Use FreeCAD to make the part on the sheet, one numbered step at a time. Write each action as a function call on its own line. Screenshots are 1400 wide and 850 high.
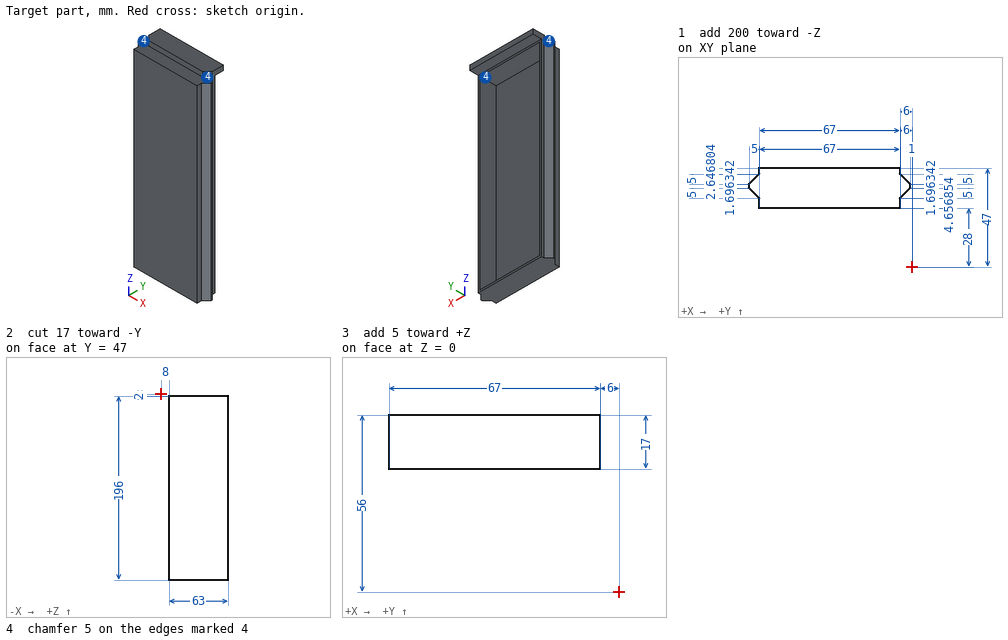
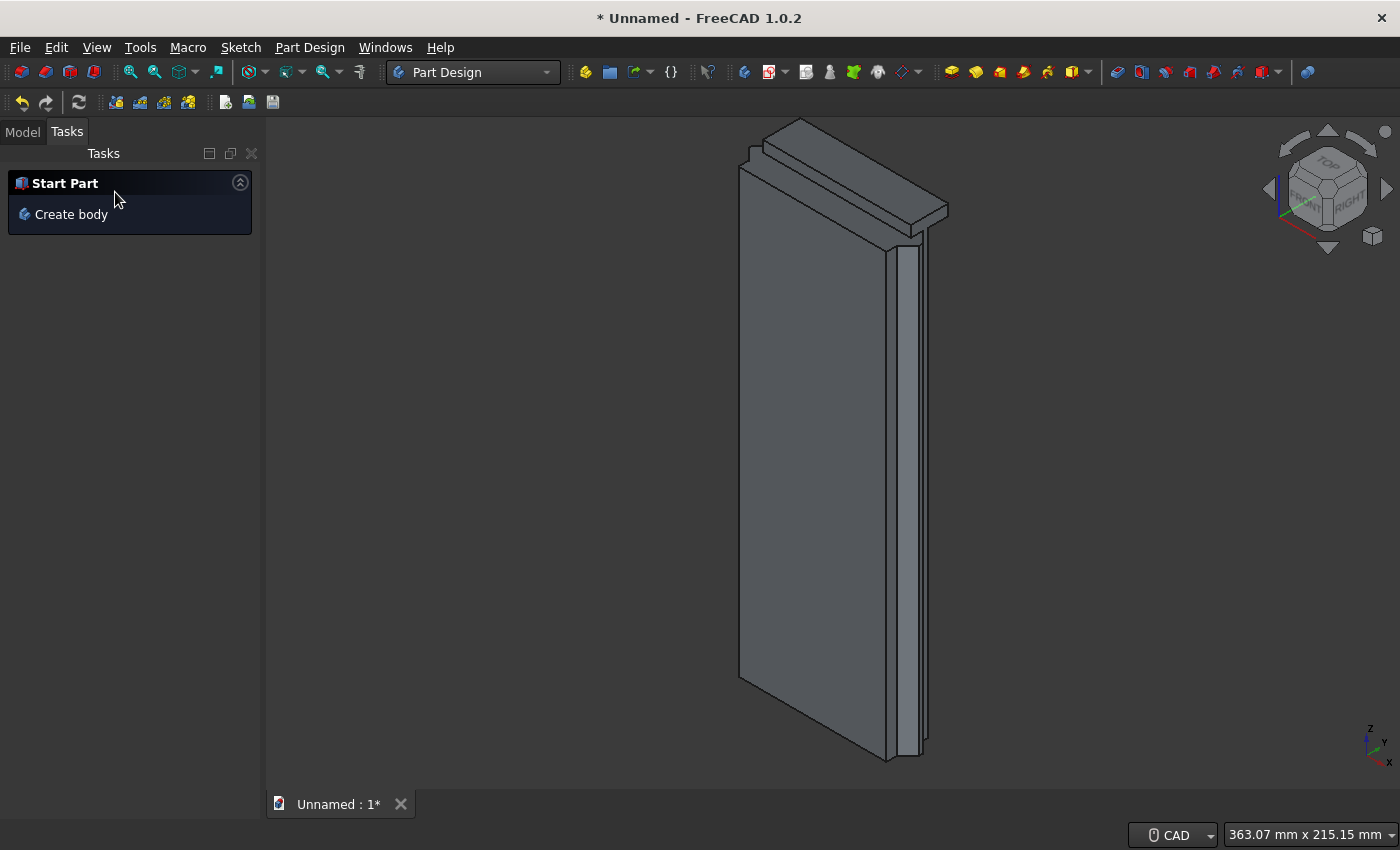
key(v)
key(f)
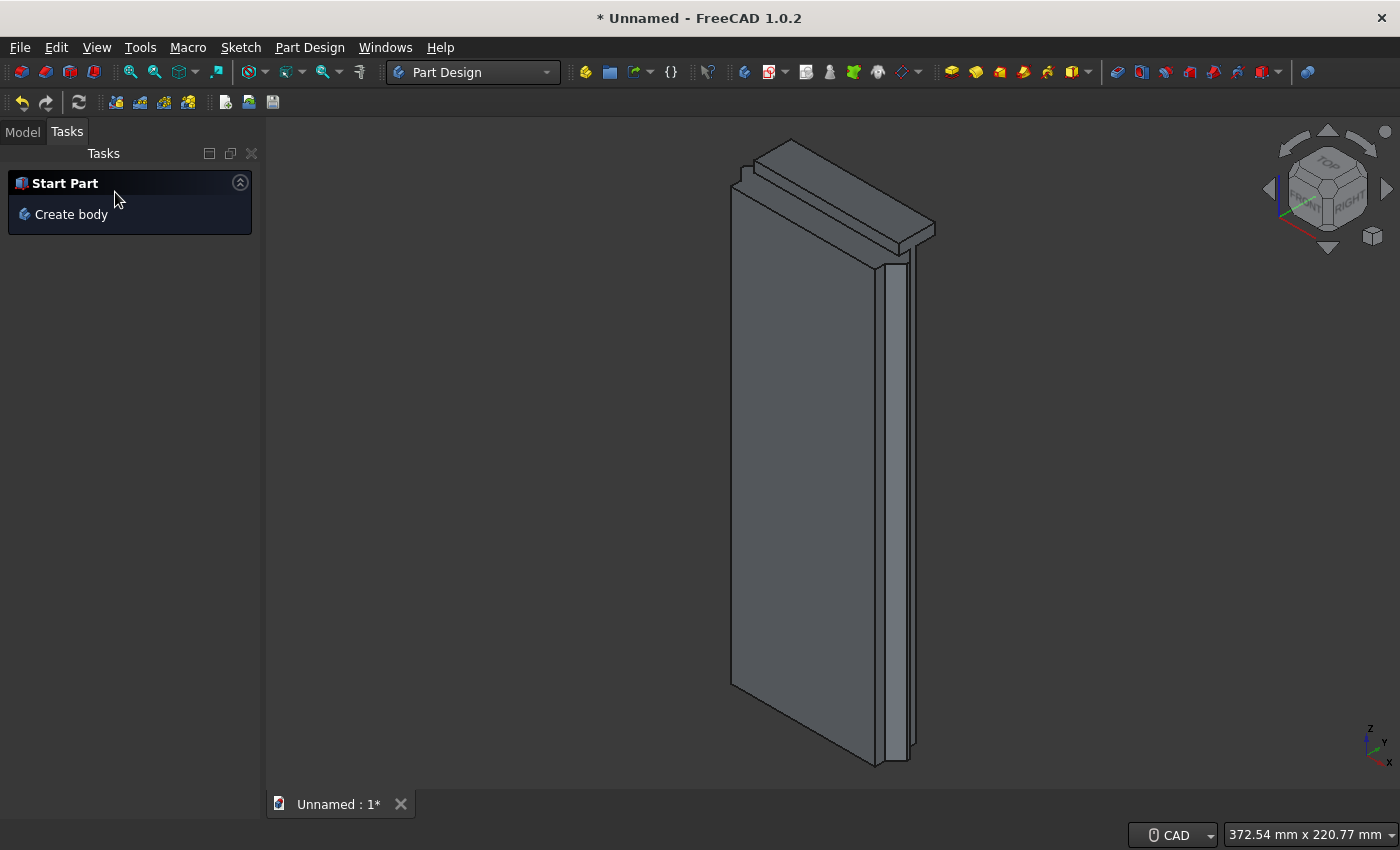
click(899, 249)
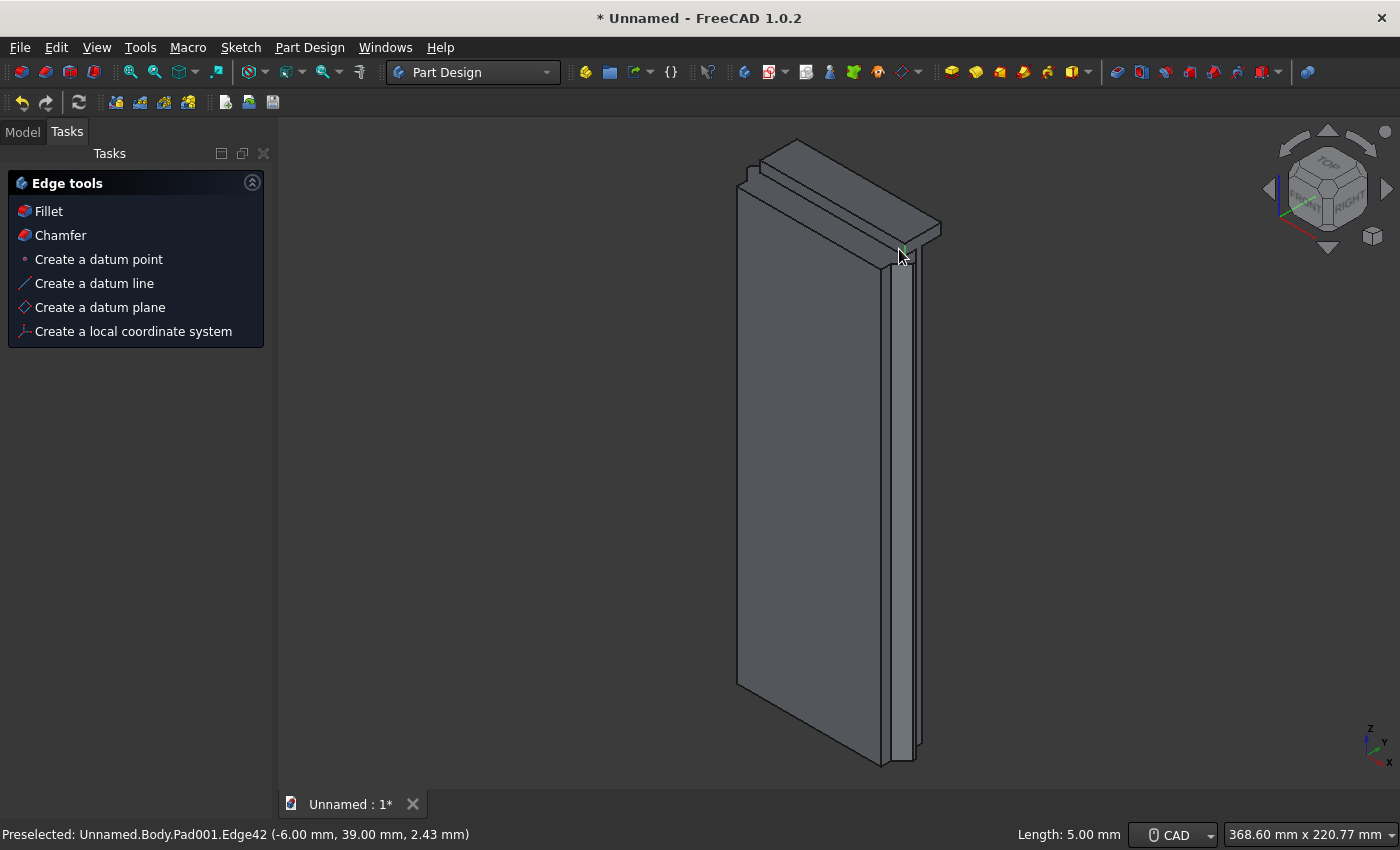
scroll(760, 166, up, 5)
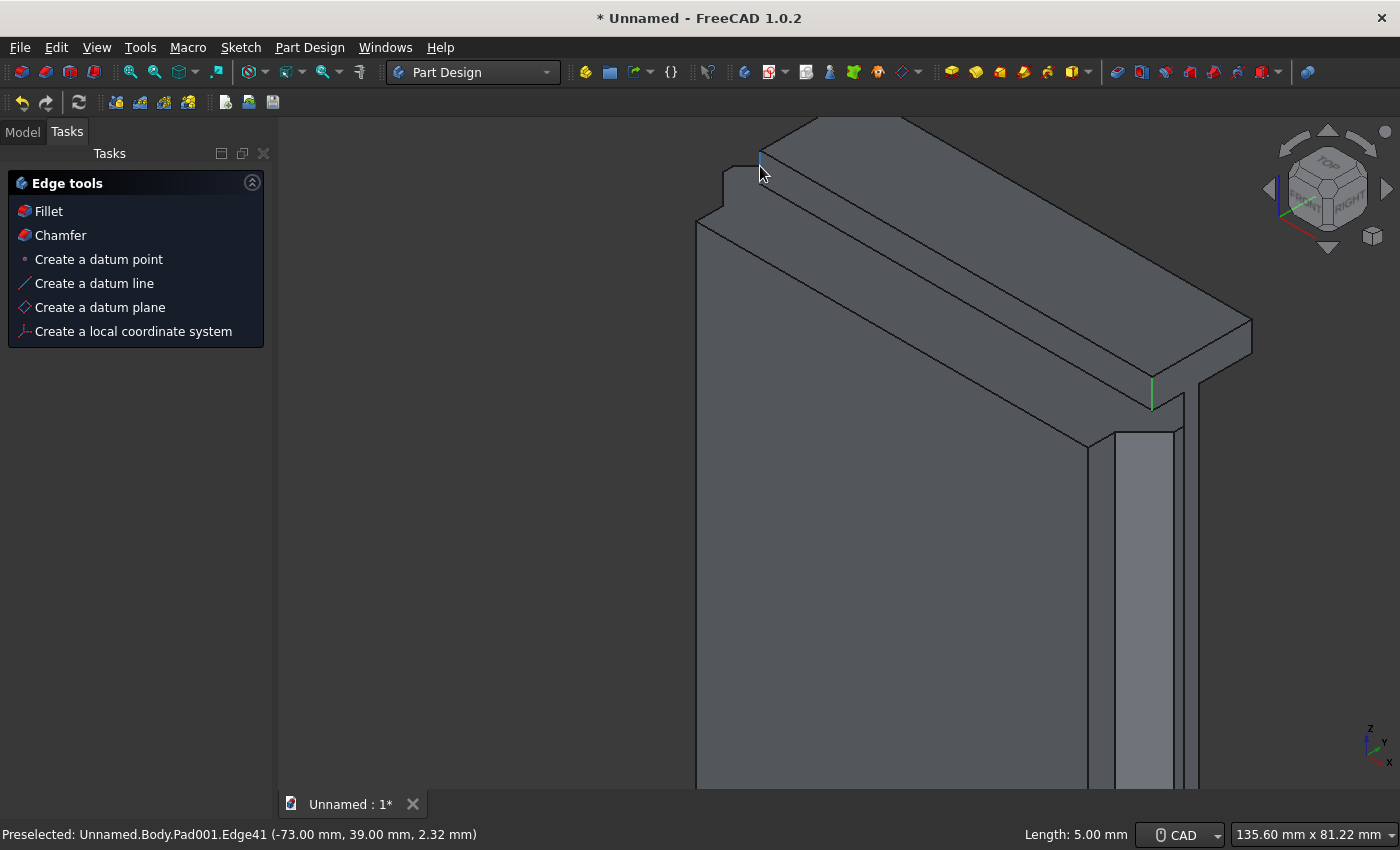
key(v)
key(f)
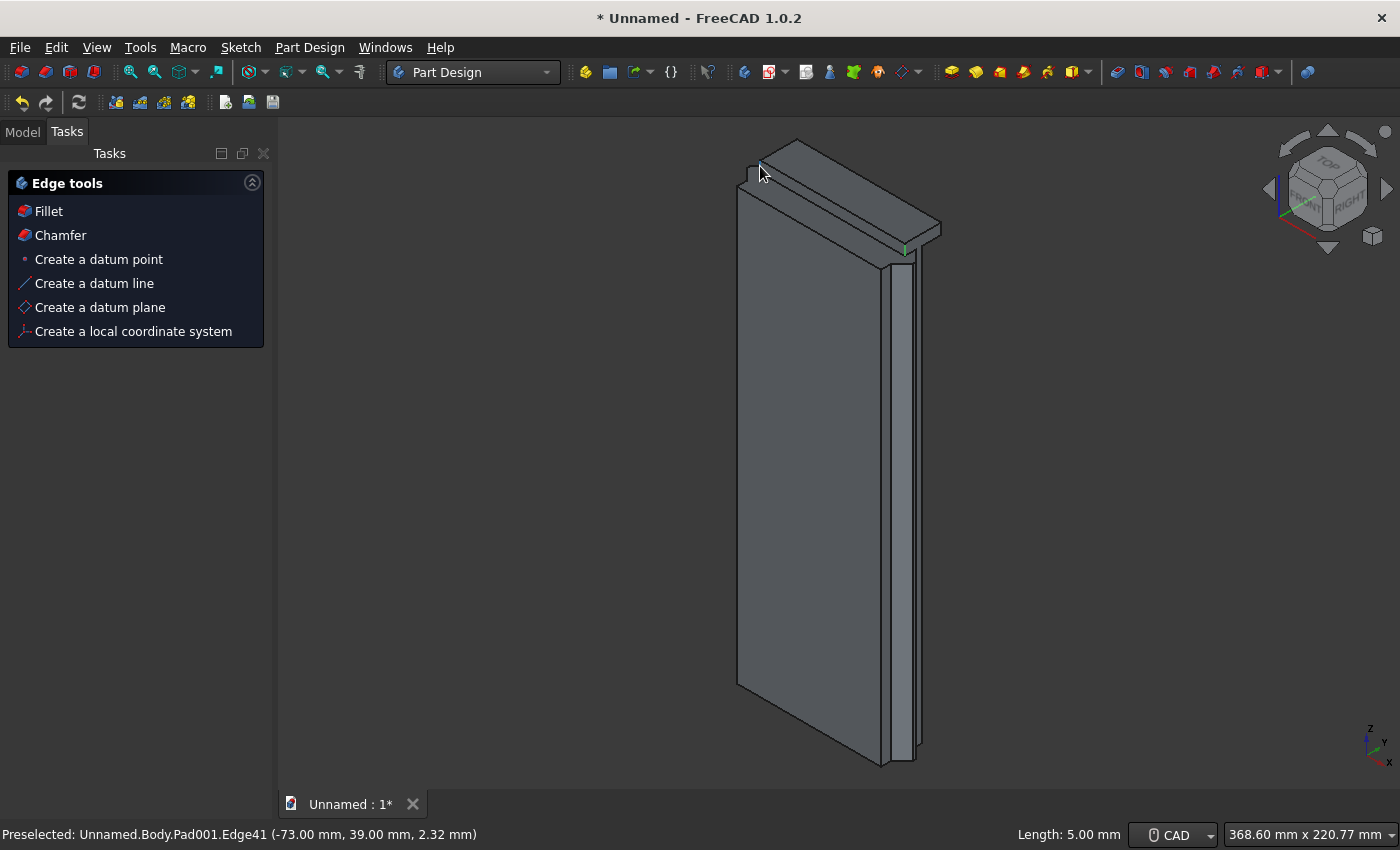
key(2)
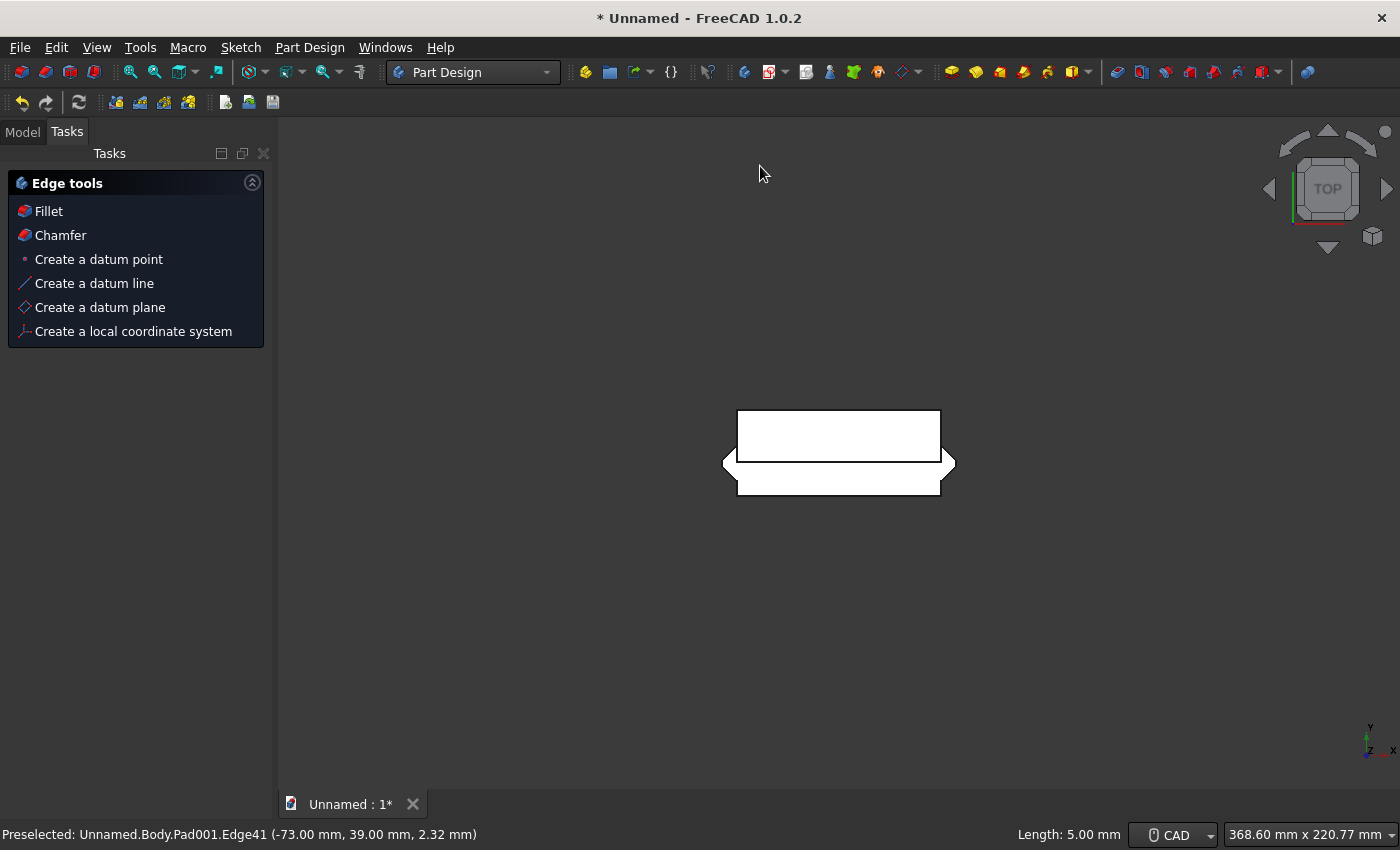
key(v)
key(f)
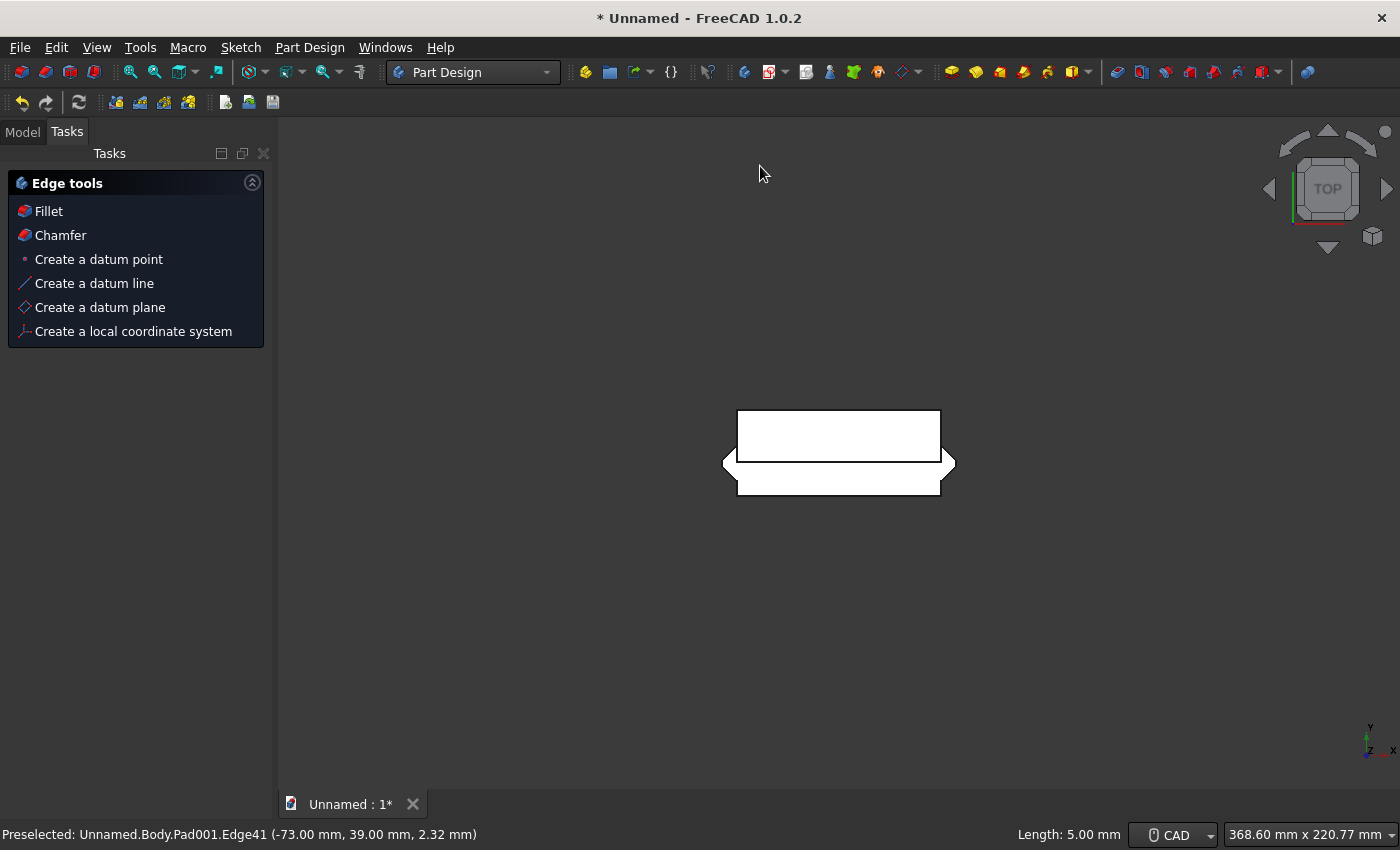
scroll(737, 461, up, 5)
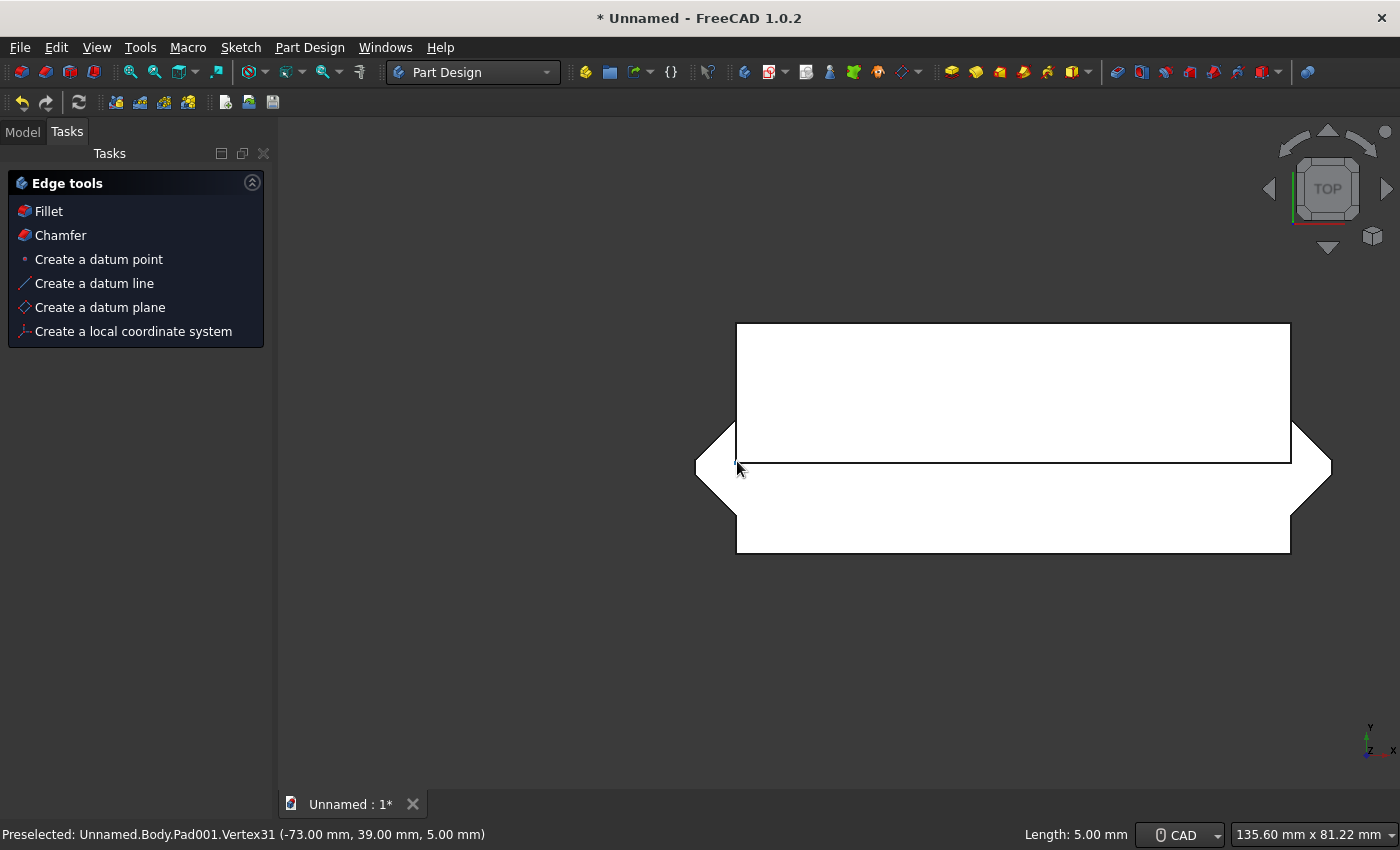
click(132, 72)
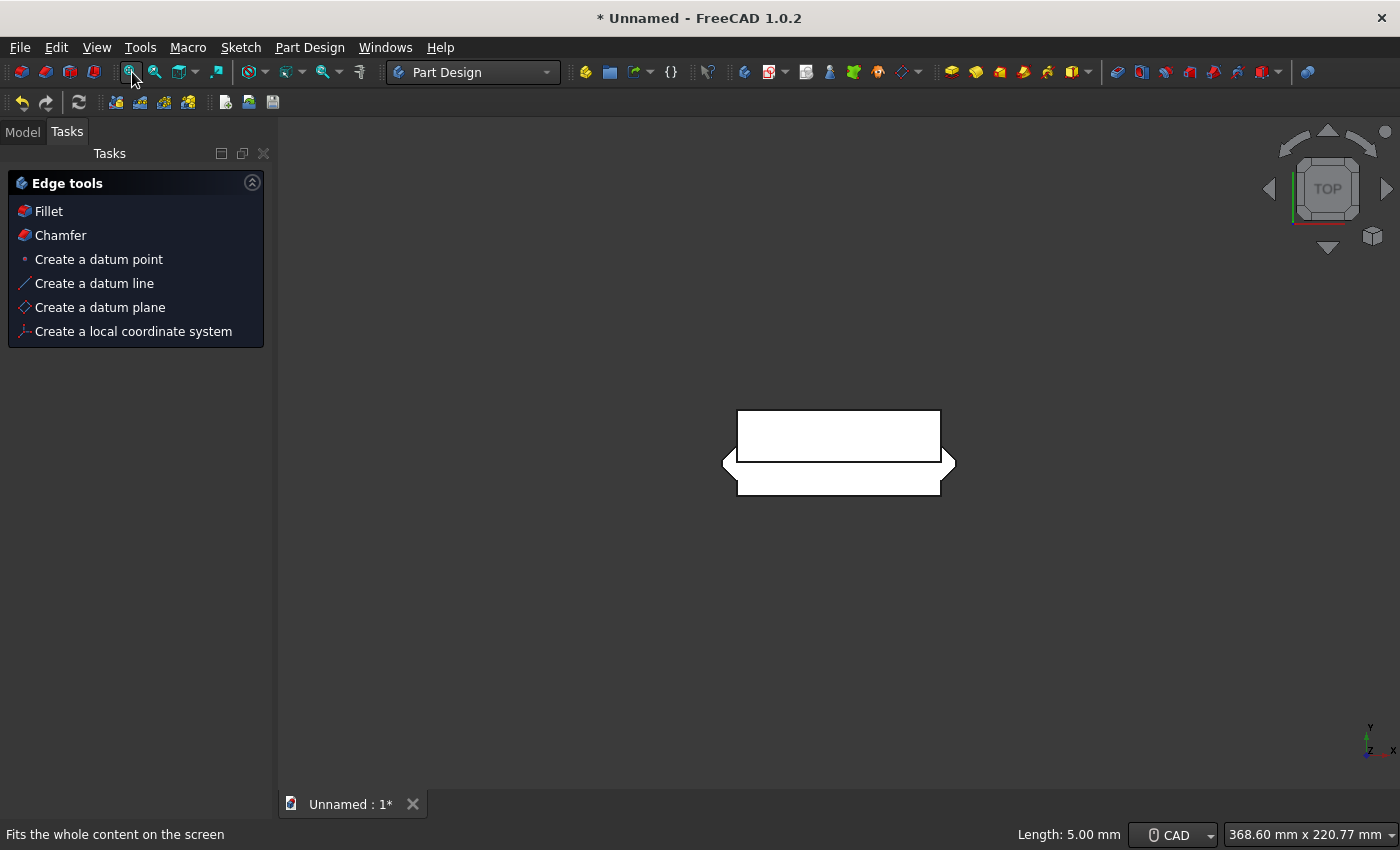
key(0)